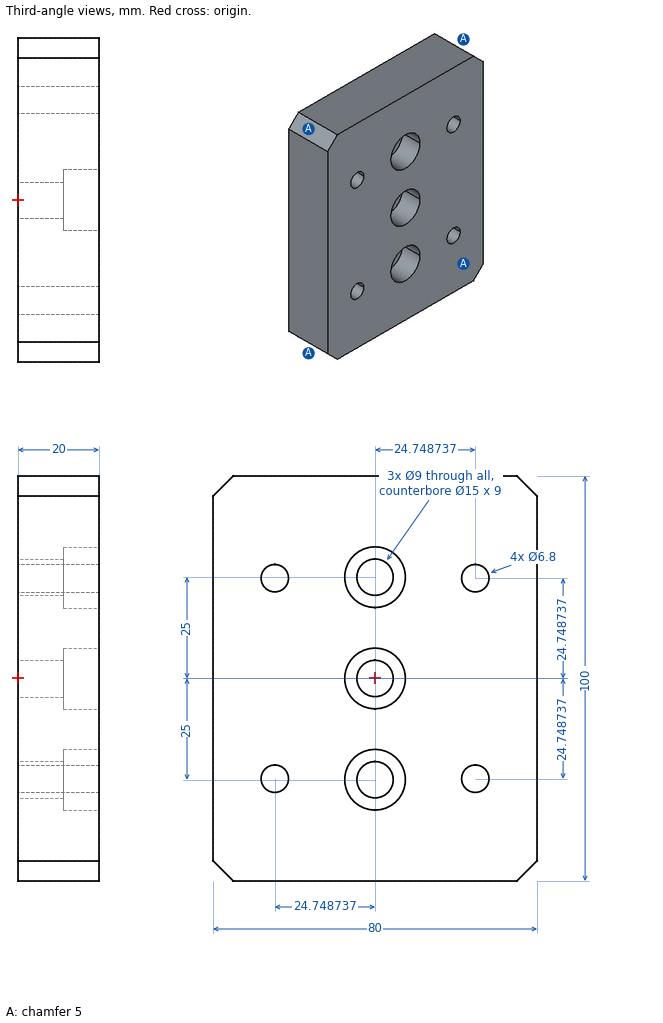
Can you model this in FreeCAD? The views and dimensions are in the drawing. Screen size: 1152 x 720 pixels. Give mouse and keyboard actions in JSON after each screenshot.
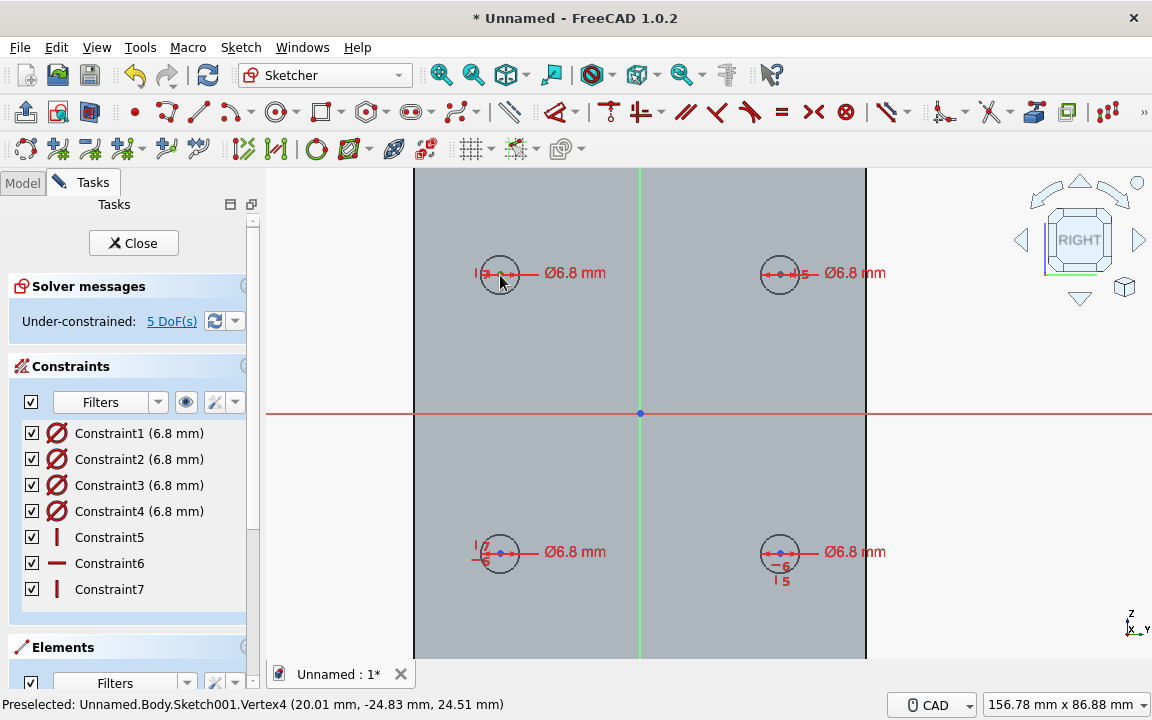
{"action": "key", "text": "h"}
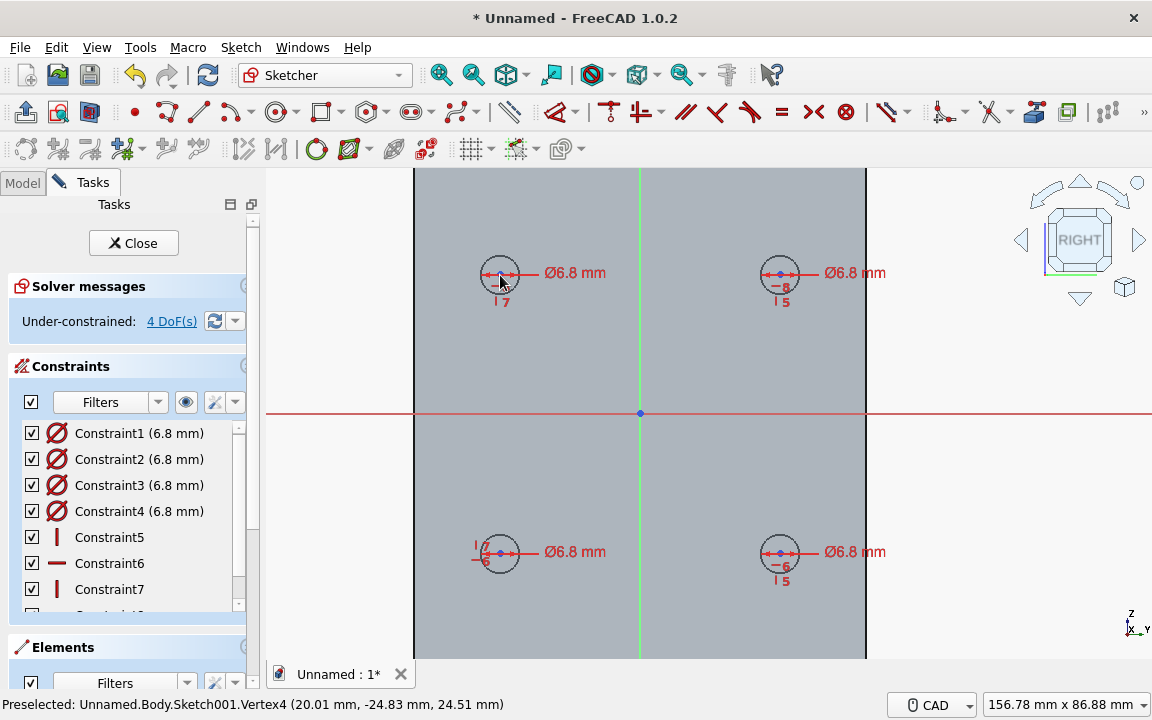
{"action": "key", "text": "d"}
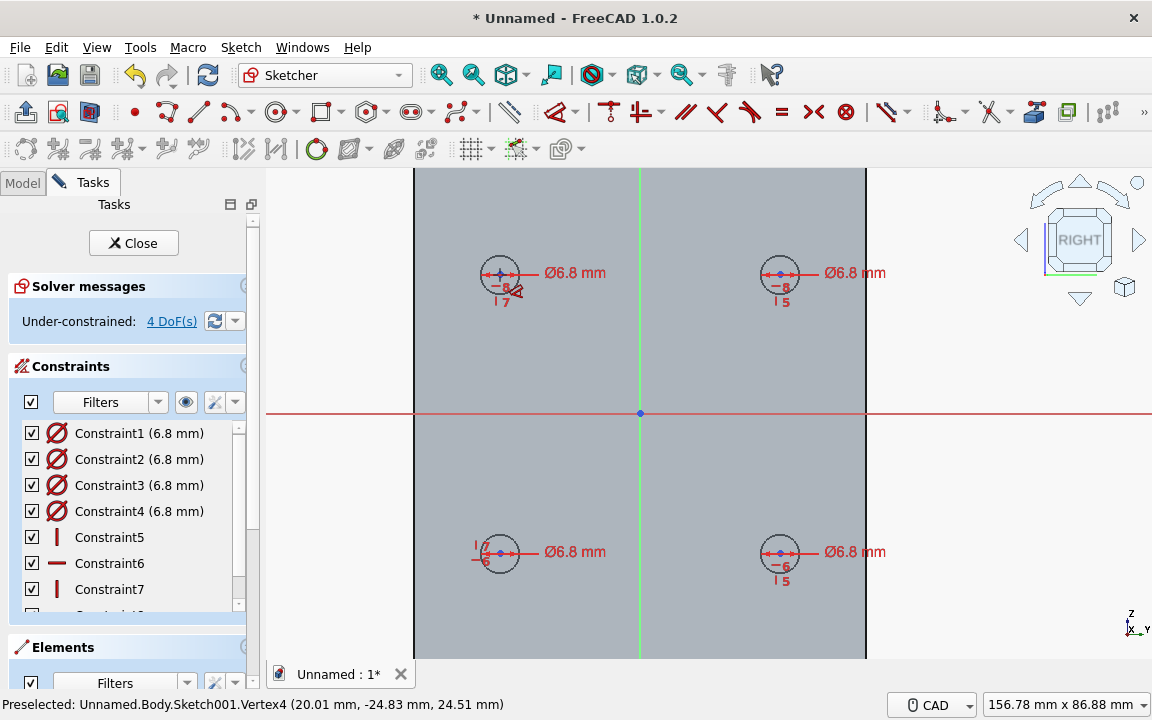
{"action": "left_click", "coordinate": [780, 275]}
{"action": "left_click", "coordinate": [710, 241]}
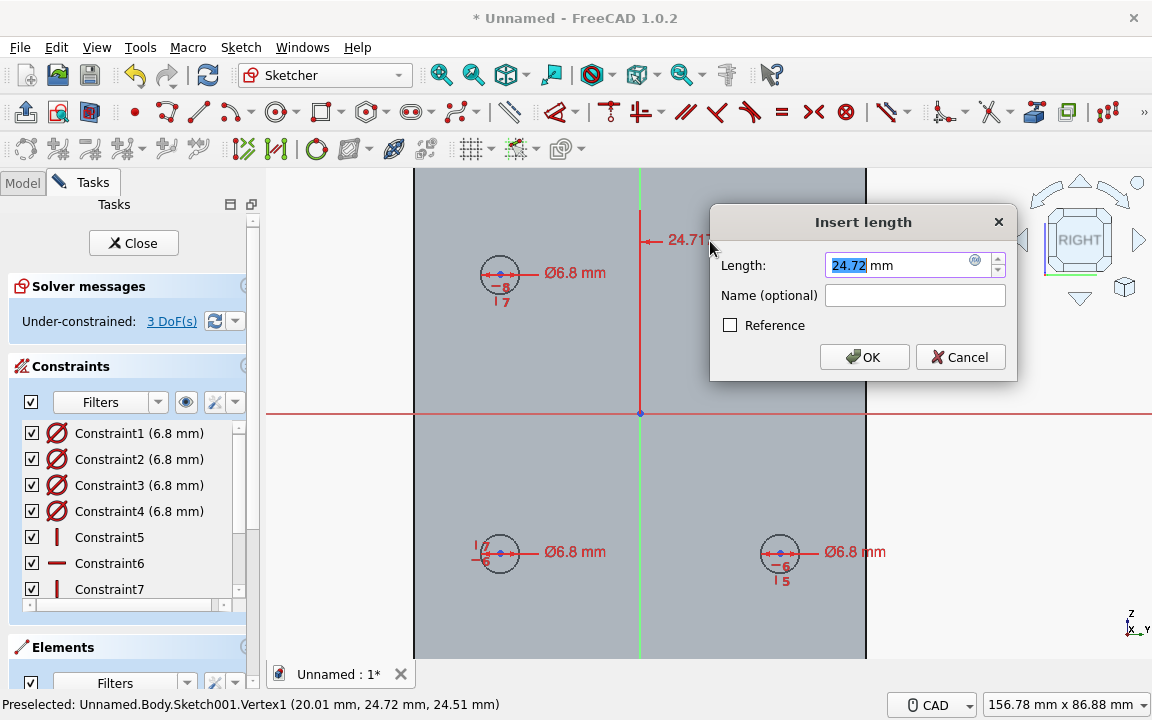
{"action": "type", "text": "24.748737"}
{"action": "key", "text": "Return"}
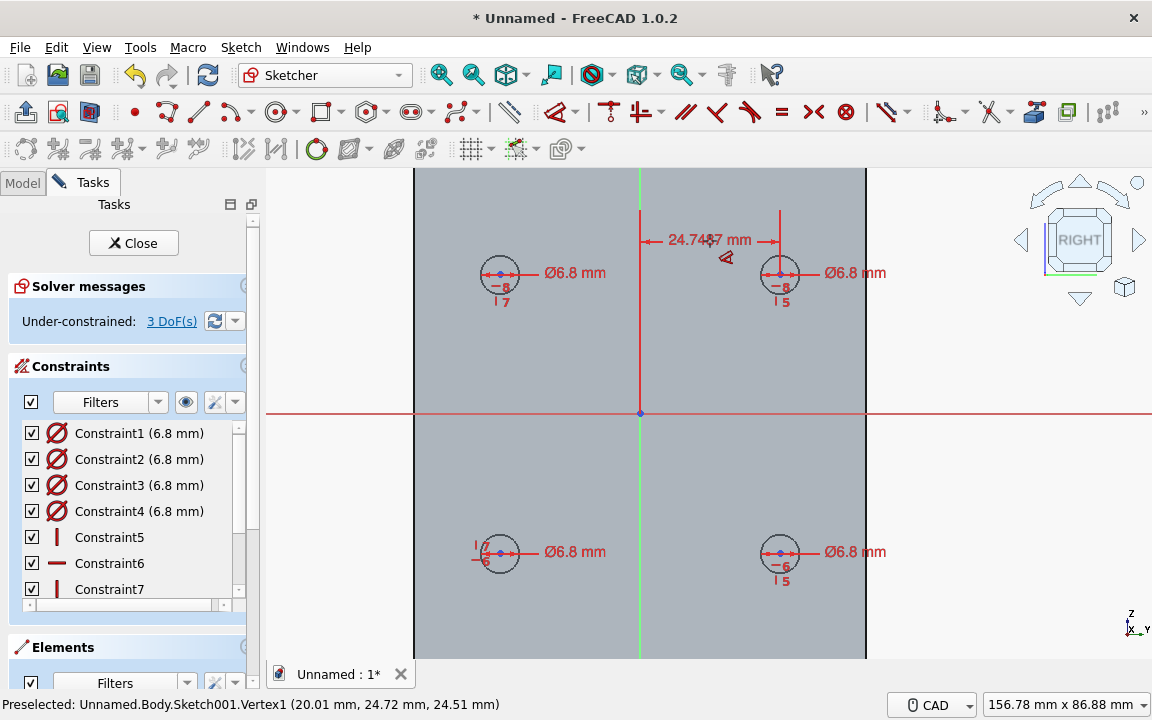
{"action": "left_click", "coordinate": [780, 275]}
{"action": "left_click", "coordinate": [814, 344]}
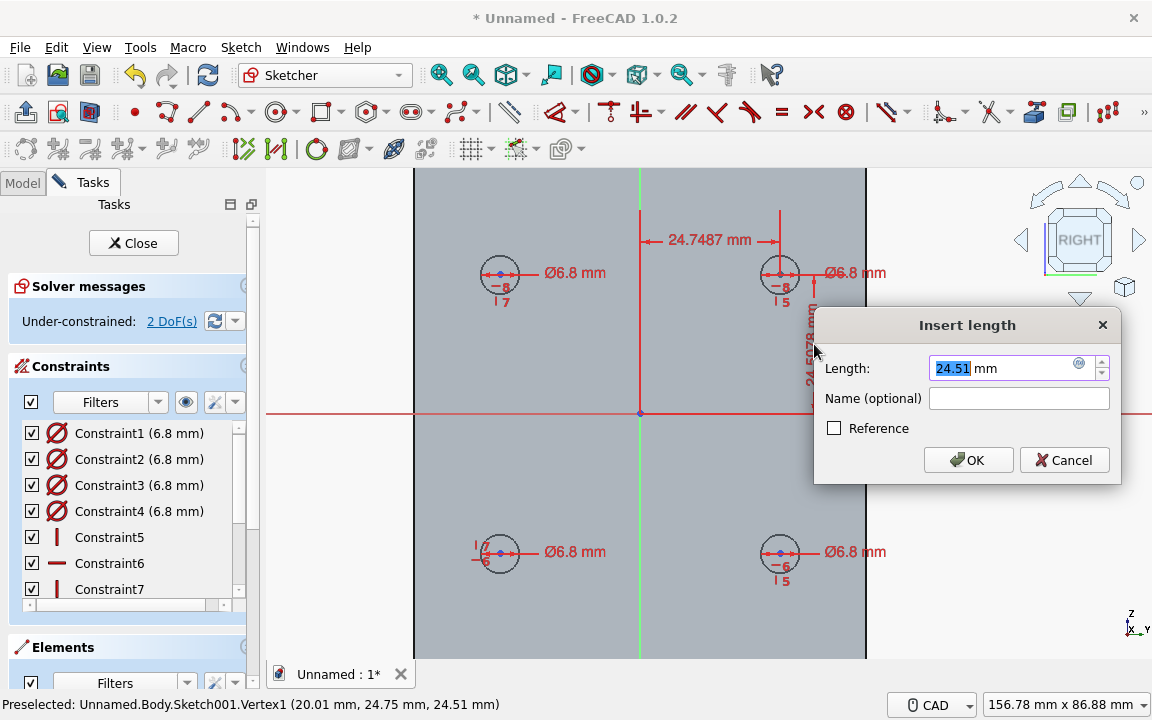
{"action": "type", "text": "24.748737"}
{"action": "key", "text": "Return"}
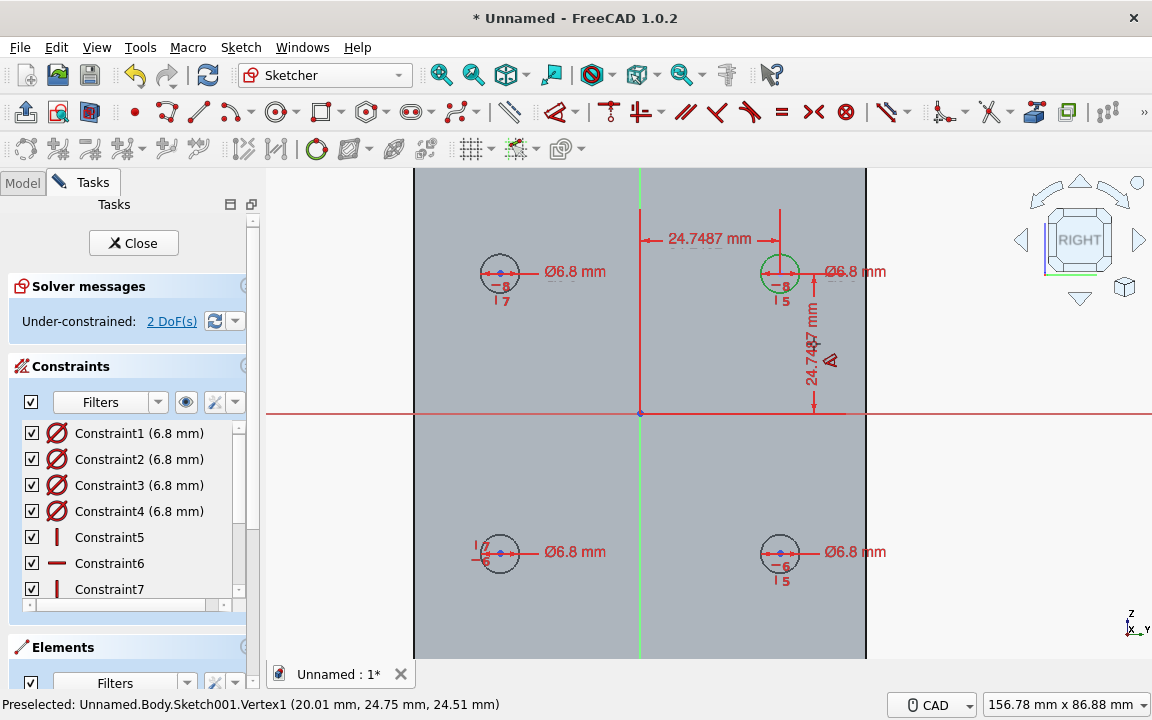
{"action": "left_click", "coordinate": [780, 554]}
{"action": "left_click", "coordinate": [814, 484]}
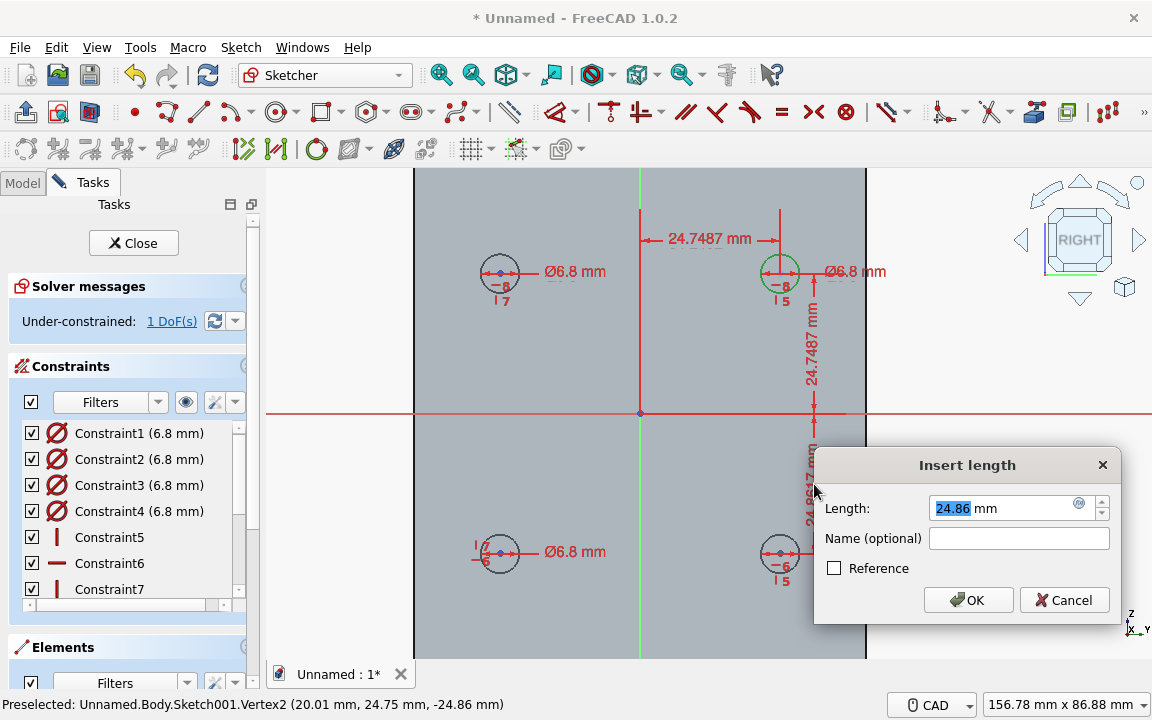
{"action": "type", "text": "24.748737"}
{"action": "key", "text": "Return"}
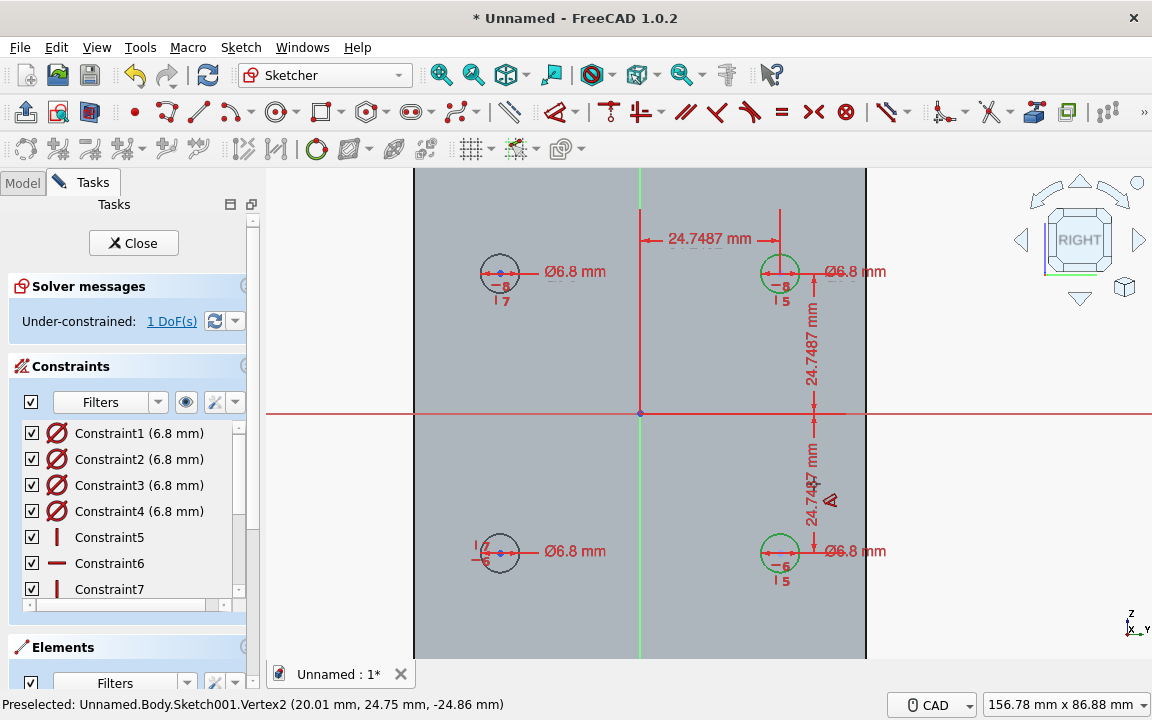
{"action": "left_click", "coordinate": [500, 553]}
{"action": "left_click", "coordinate": [570, 587]}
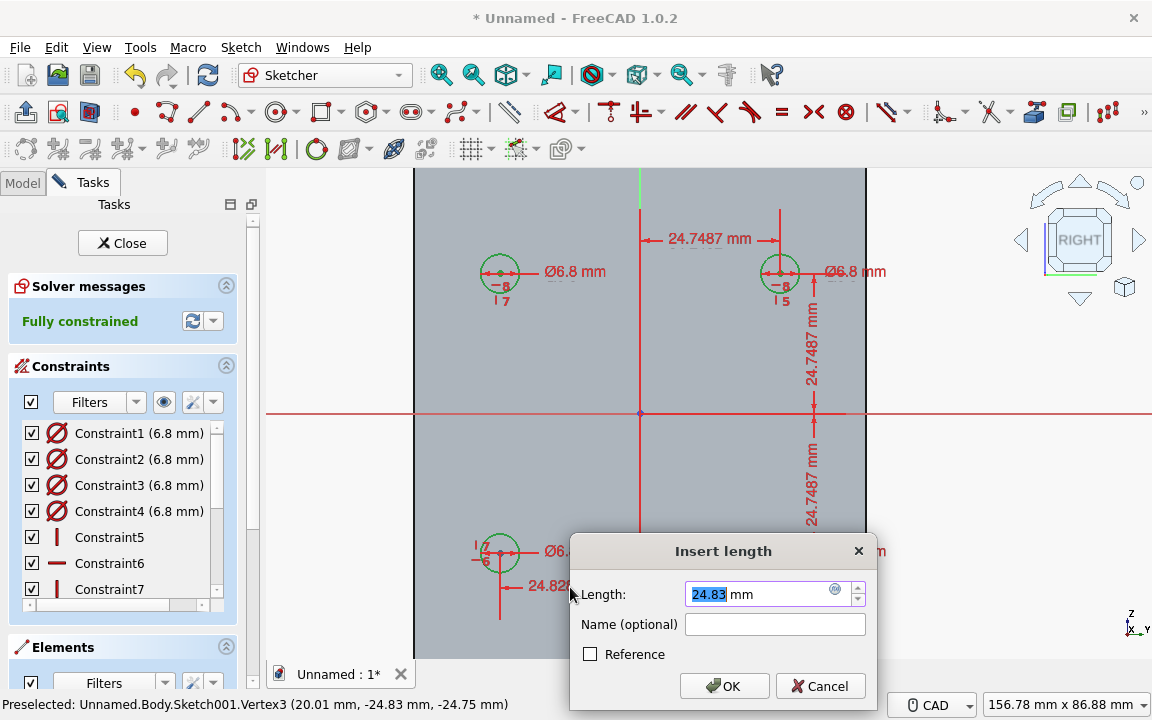
{"action": "type", "text": "24.748737"}
{"action": "key", "text": "Return"}
{"action": "key", "text": "Escape"}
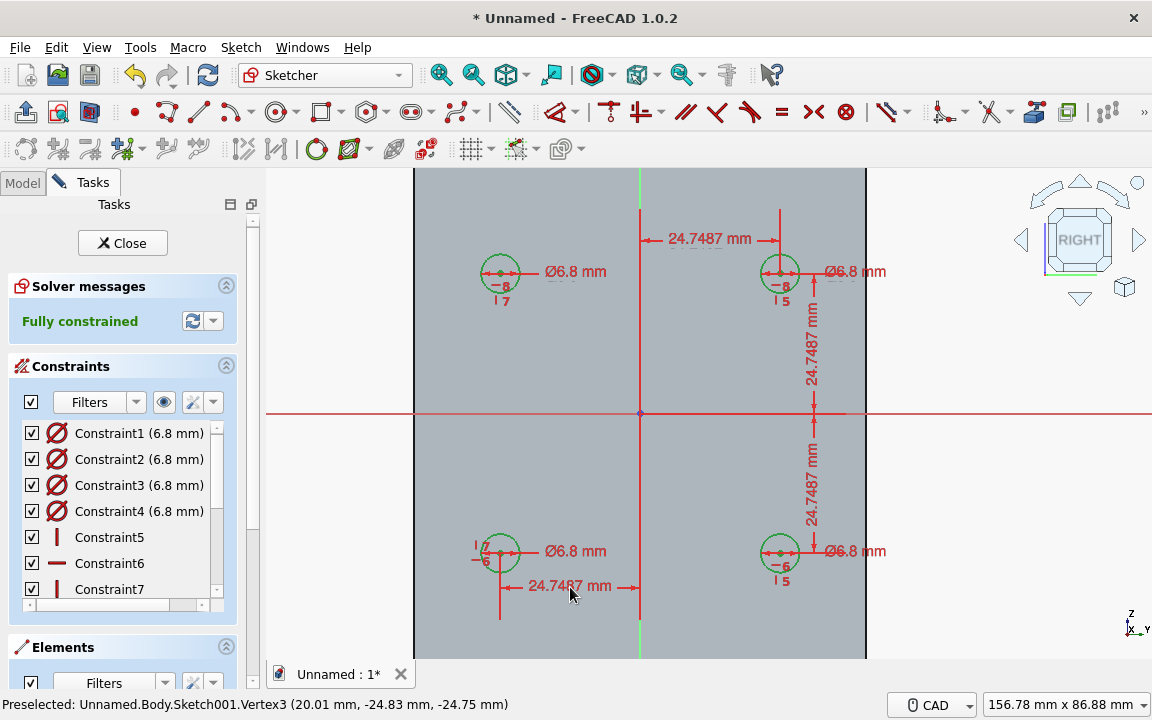
{"action": "left_click", "coordinate": [123, 243]}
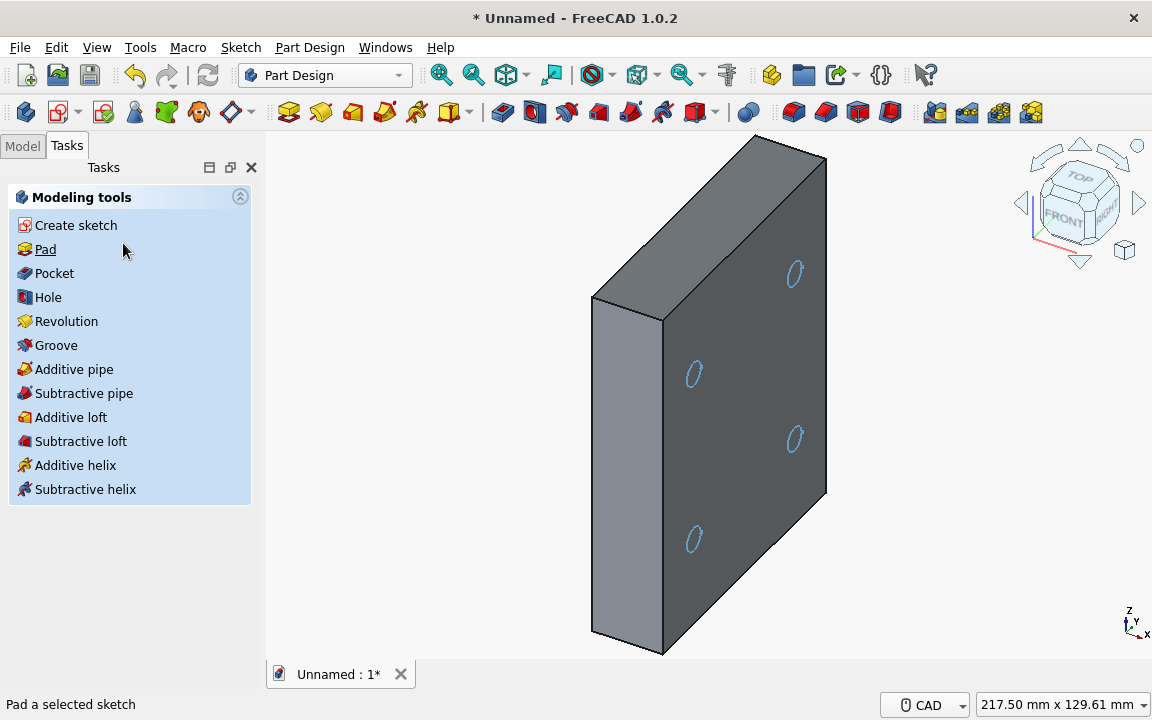
{"action": "left_click", "coordinate": [504, 112]}